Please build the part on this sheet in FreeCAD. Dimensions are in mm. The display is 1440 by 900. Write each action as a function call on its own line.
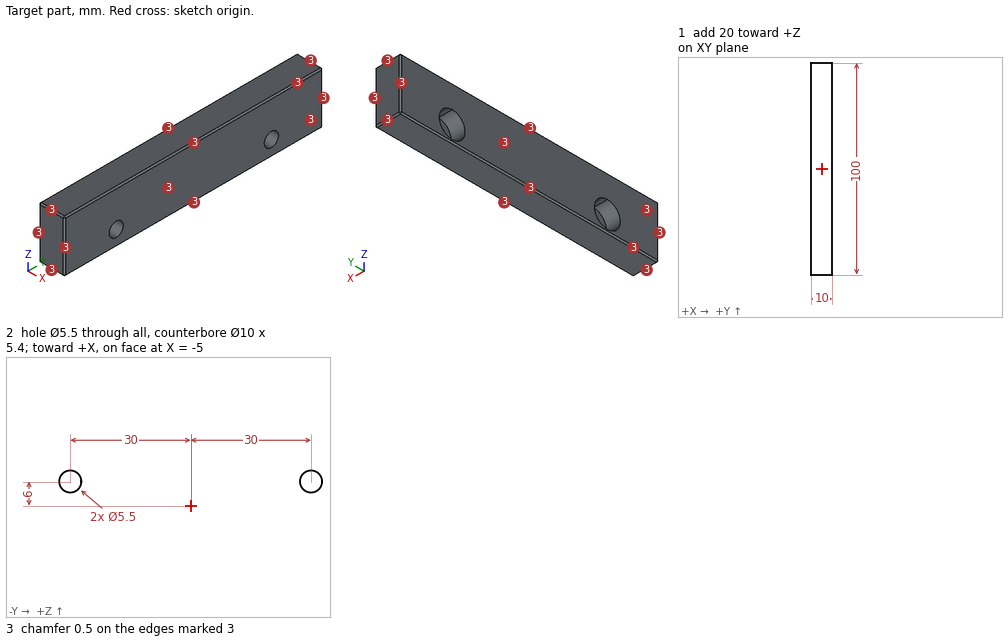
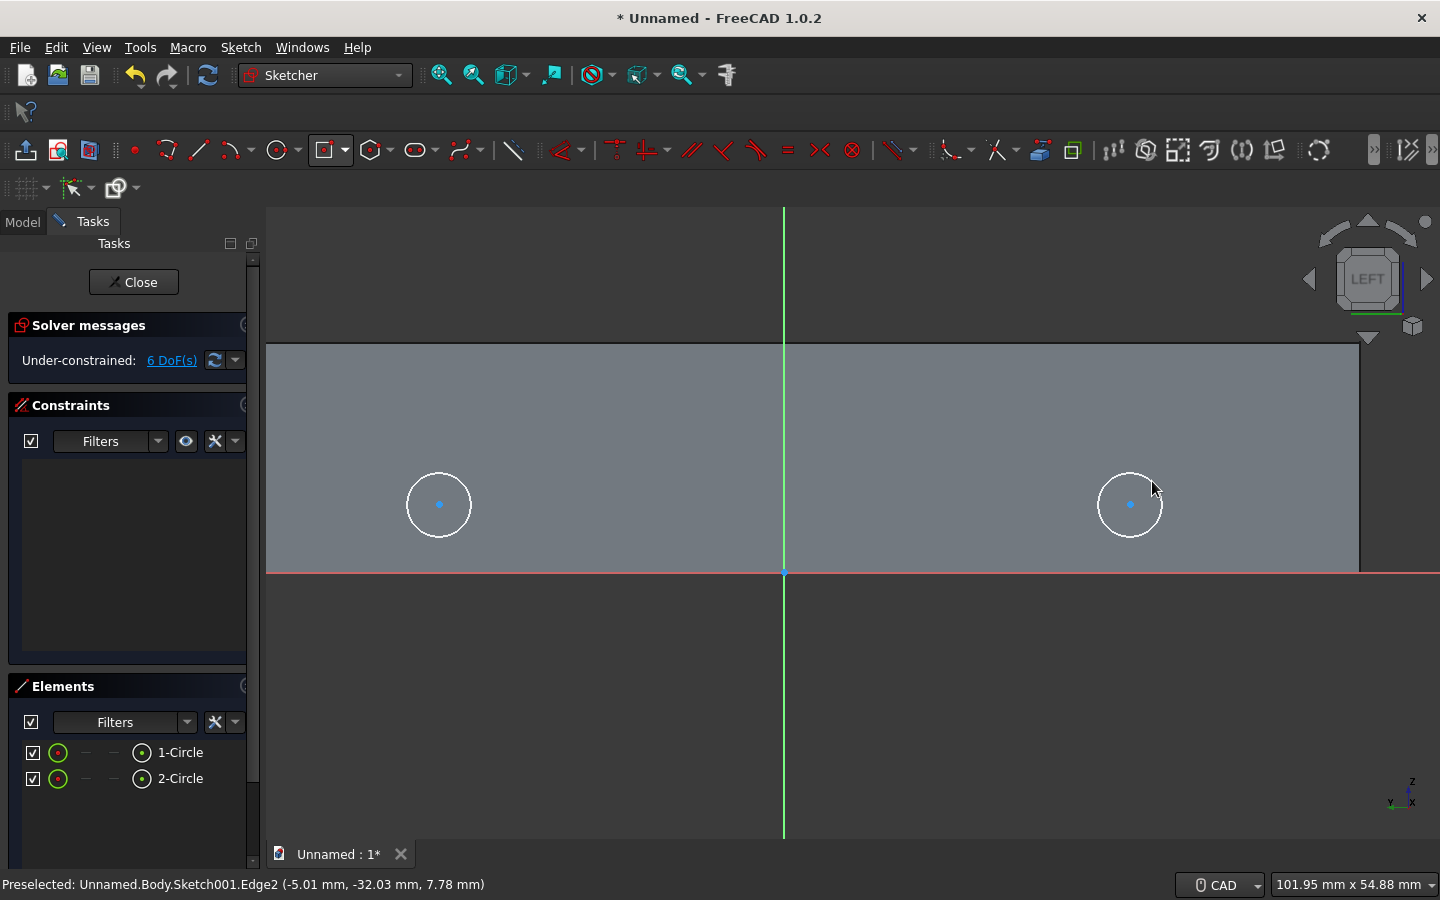
click(461, 482)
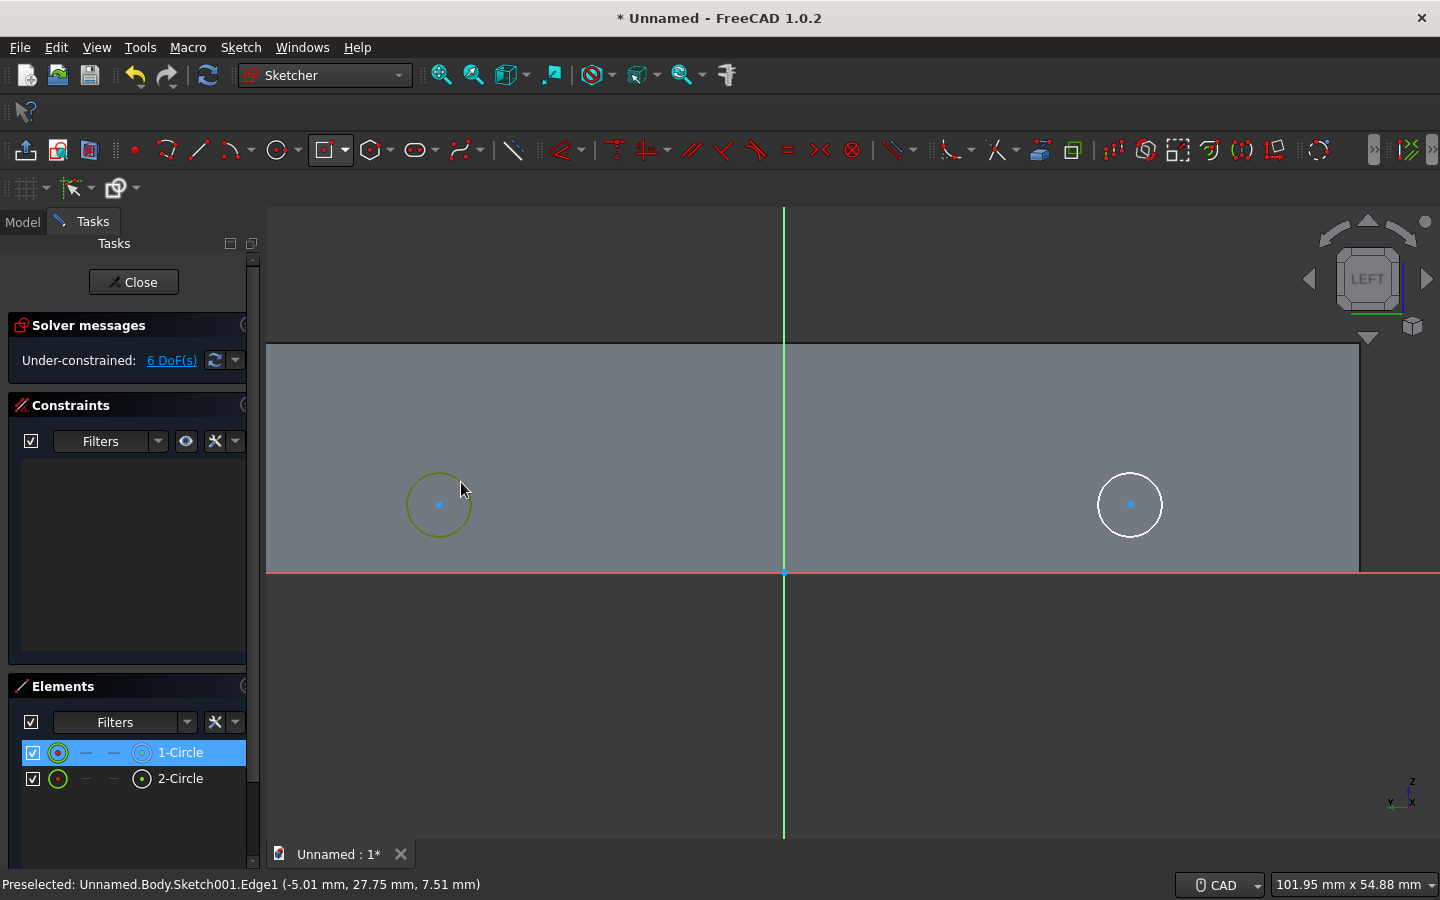
click(1152, 482)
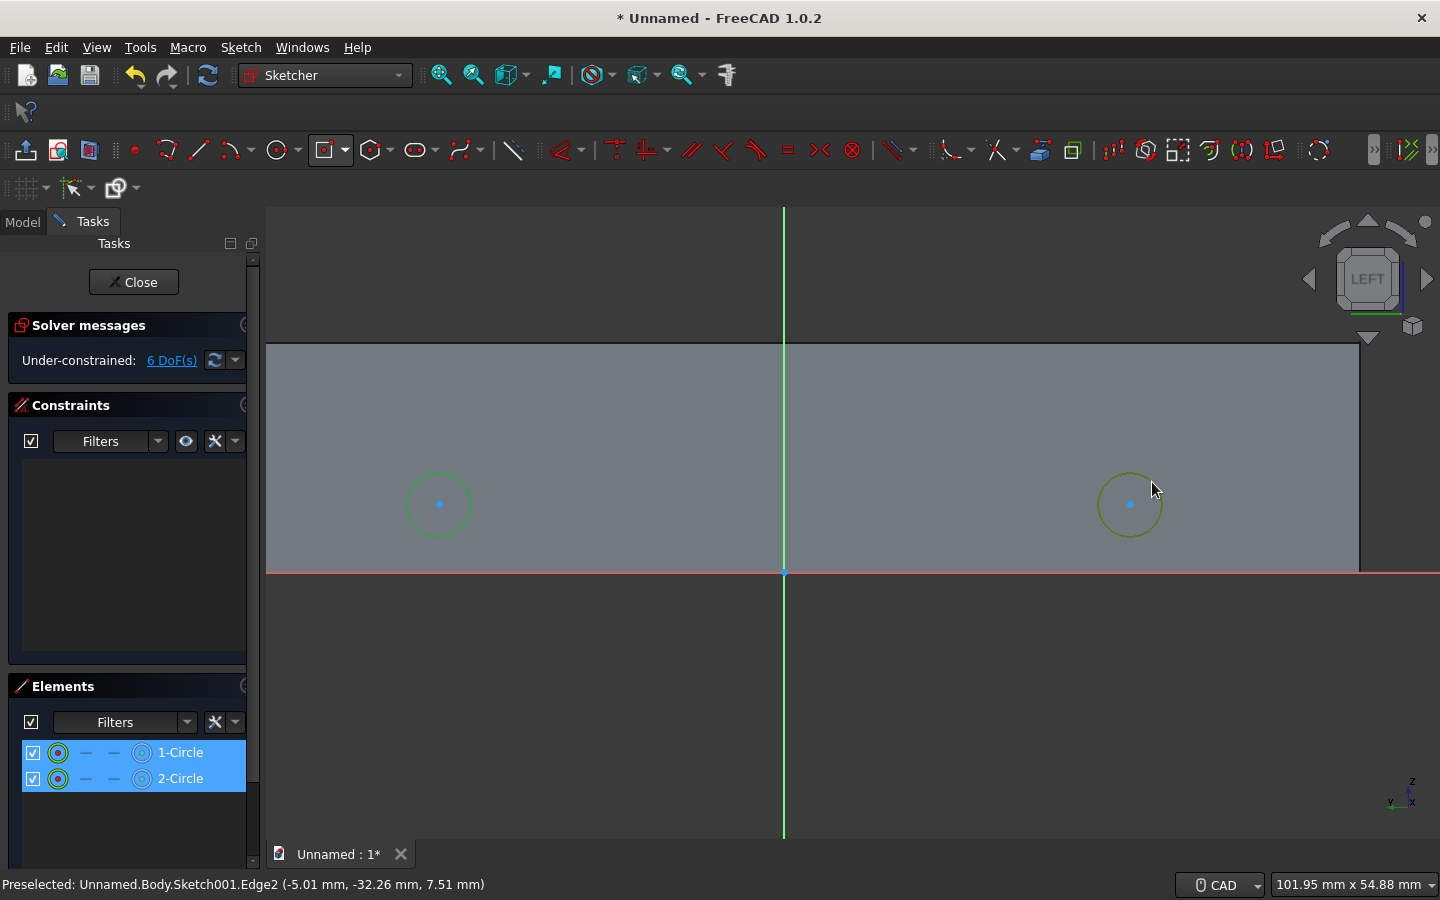
click(788, 150)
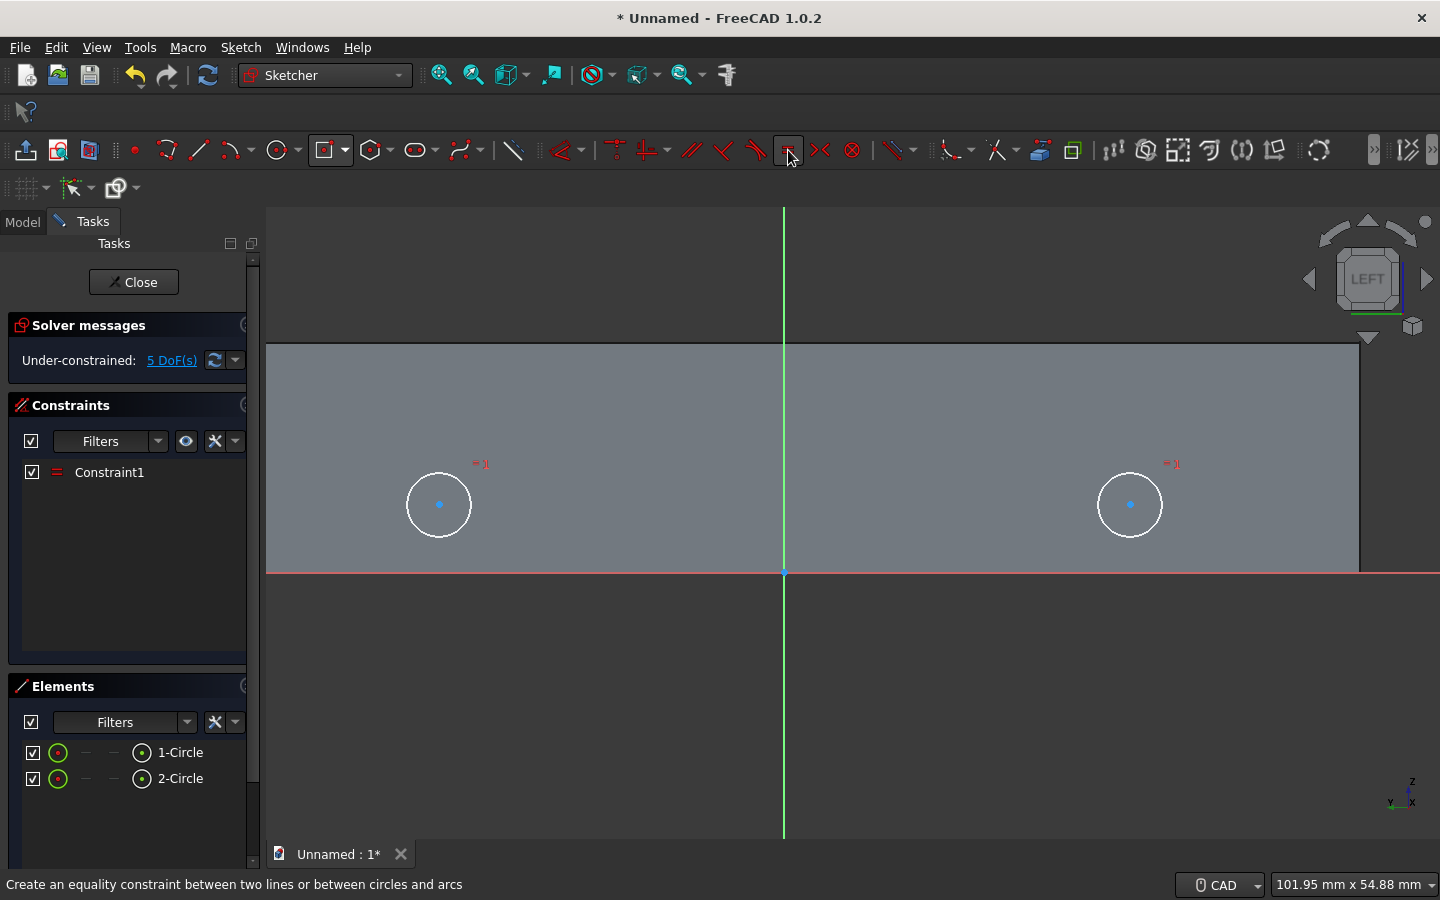
click(439, 505)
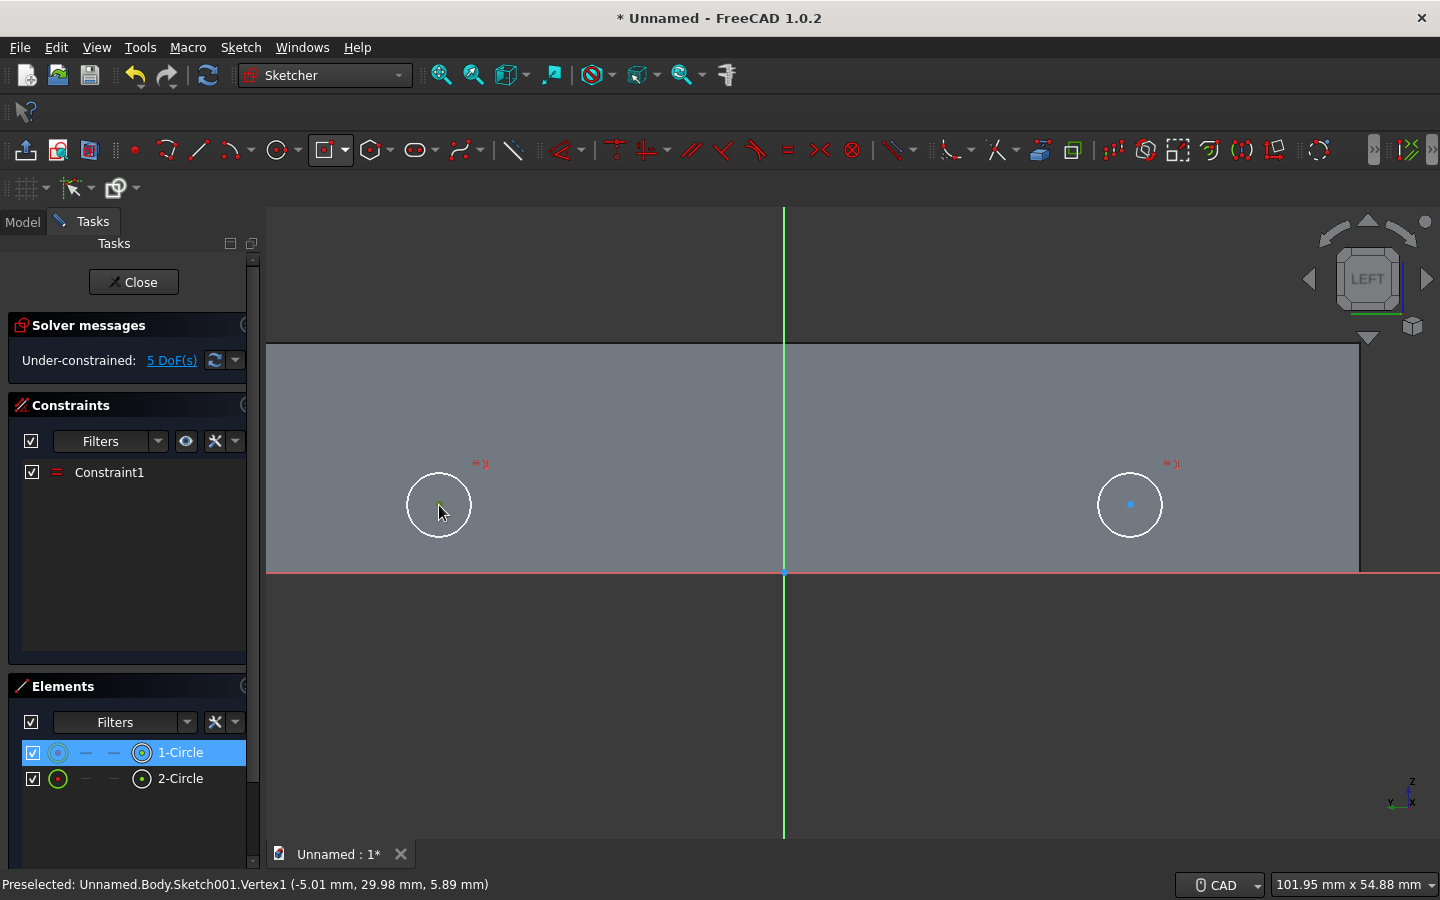
click(1130, 505)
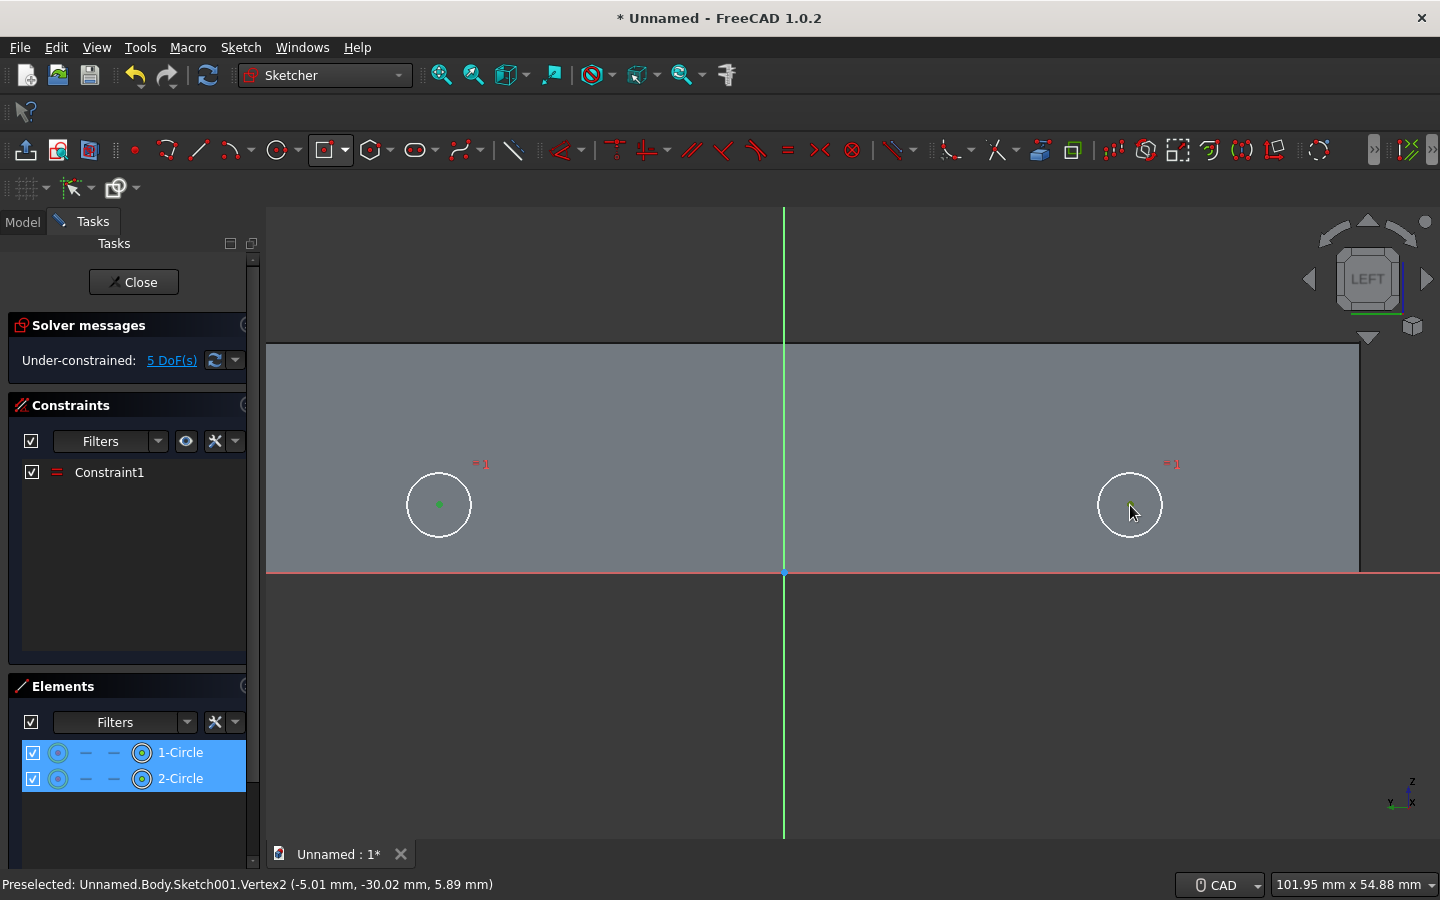
click(670, 150)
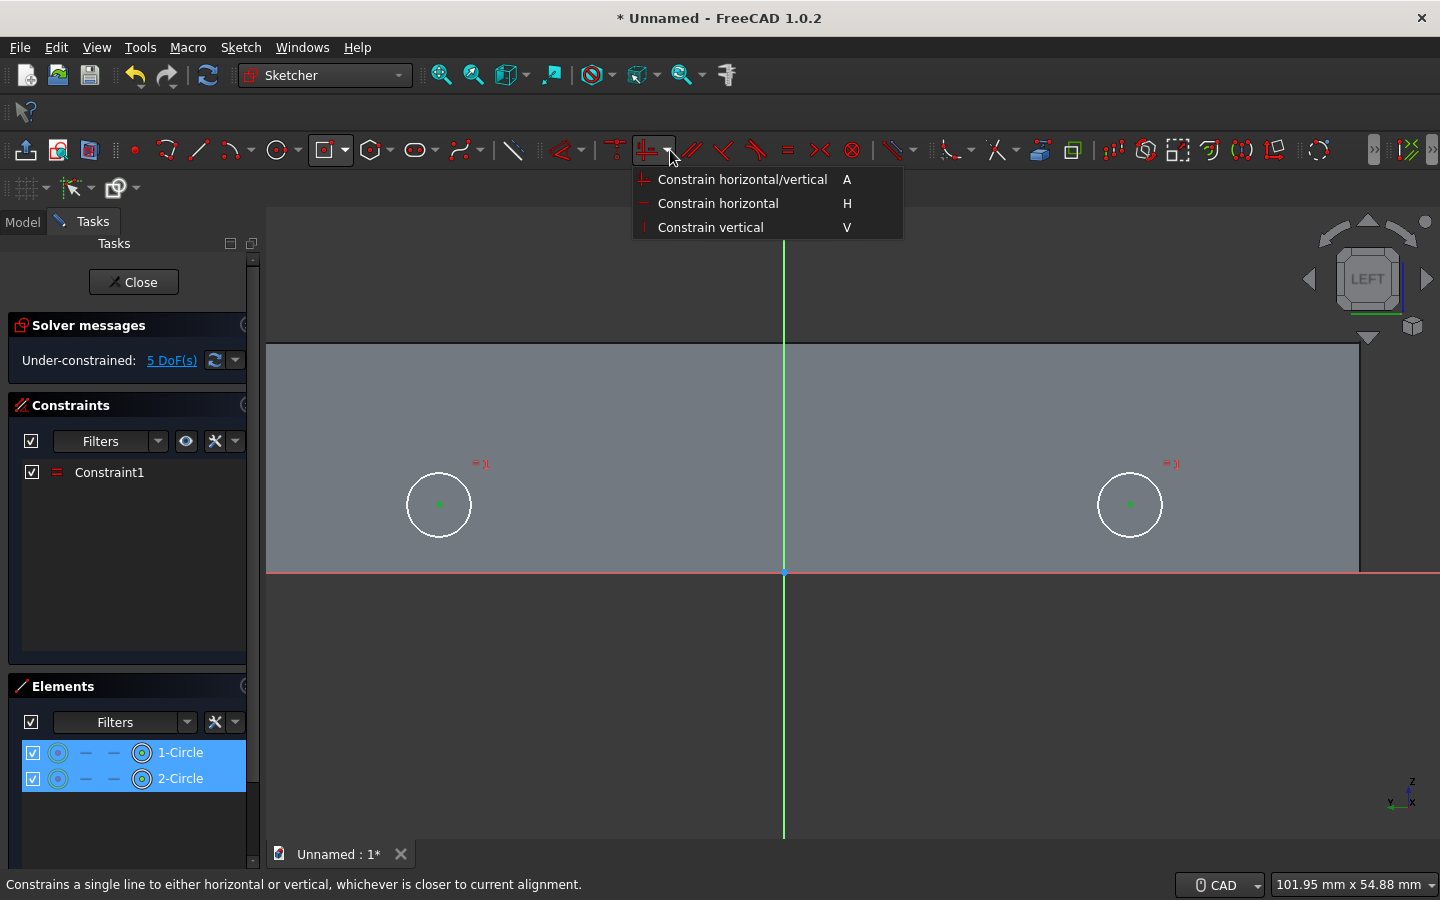
click(768, 203)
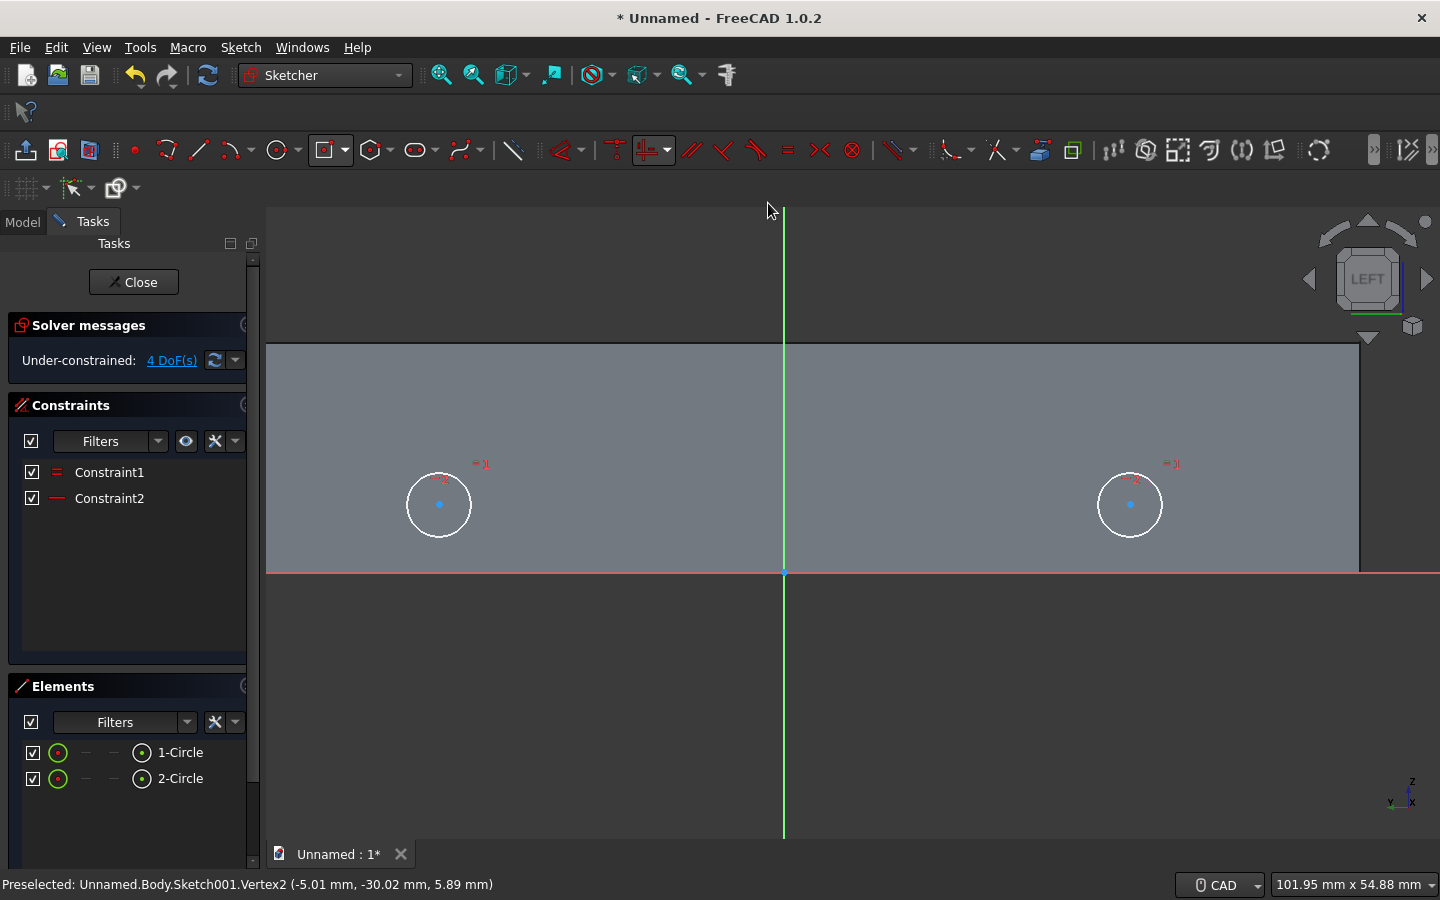
click(560, 150)